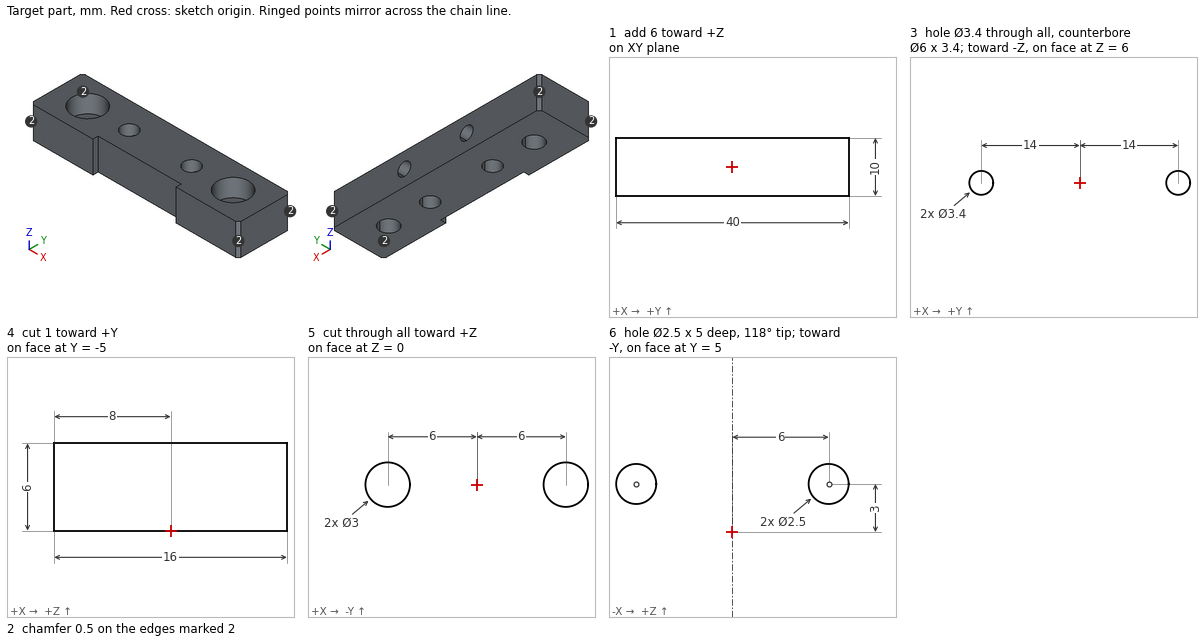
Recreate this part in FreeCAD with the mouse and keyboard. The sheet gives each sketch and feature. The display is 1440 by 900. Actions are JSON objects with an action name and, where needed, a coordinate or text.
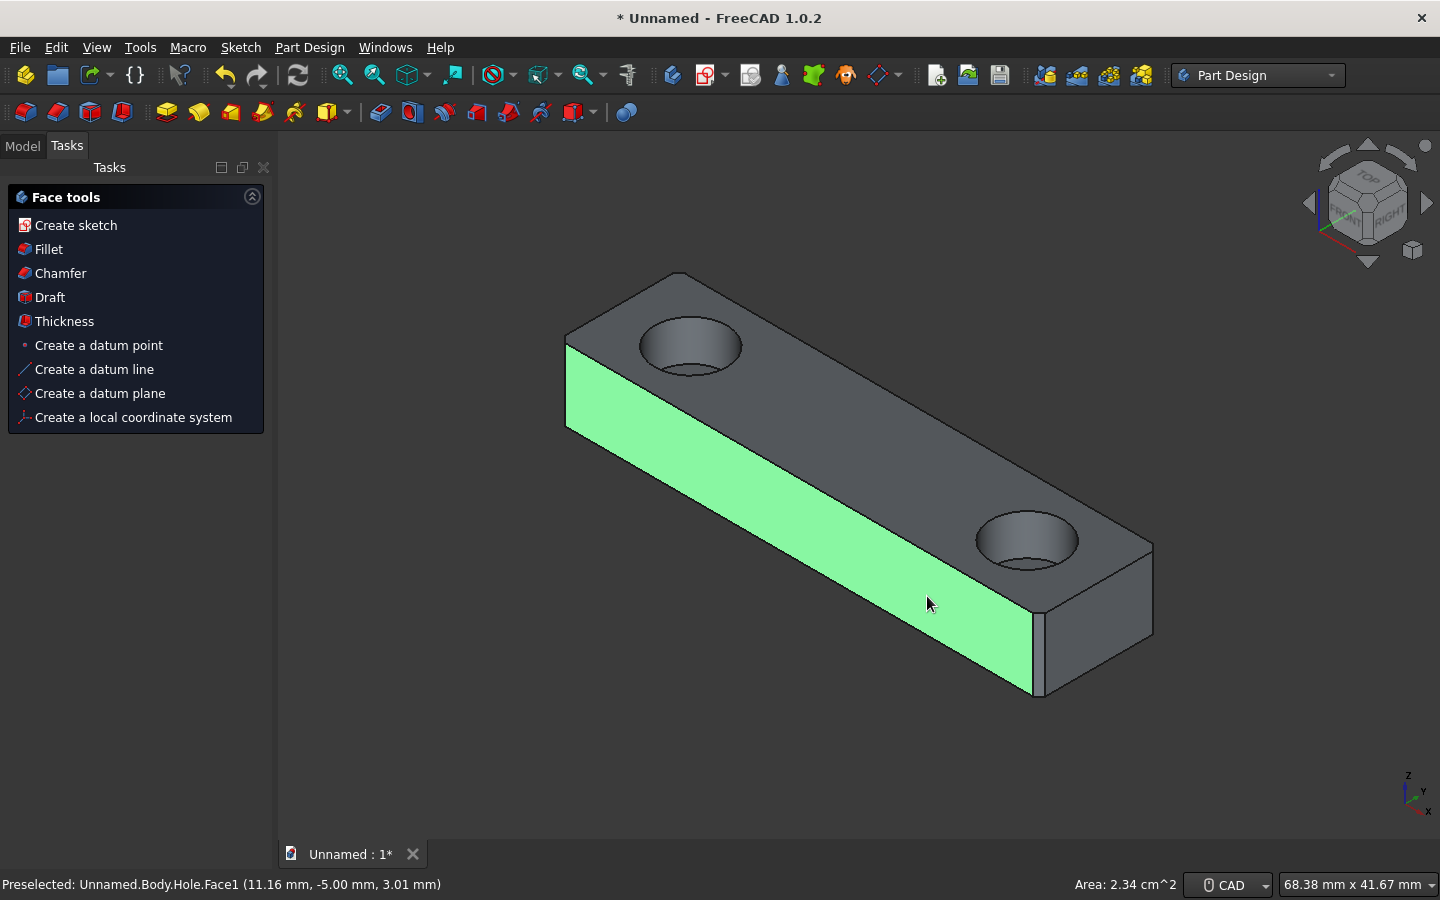
{"action": "left_click", "coordinate": [706, 76]}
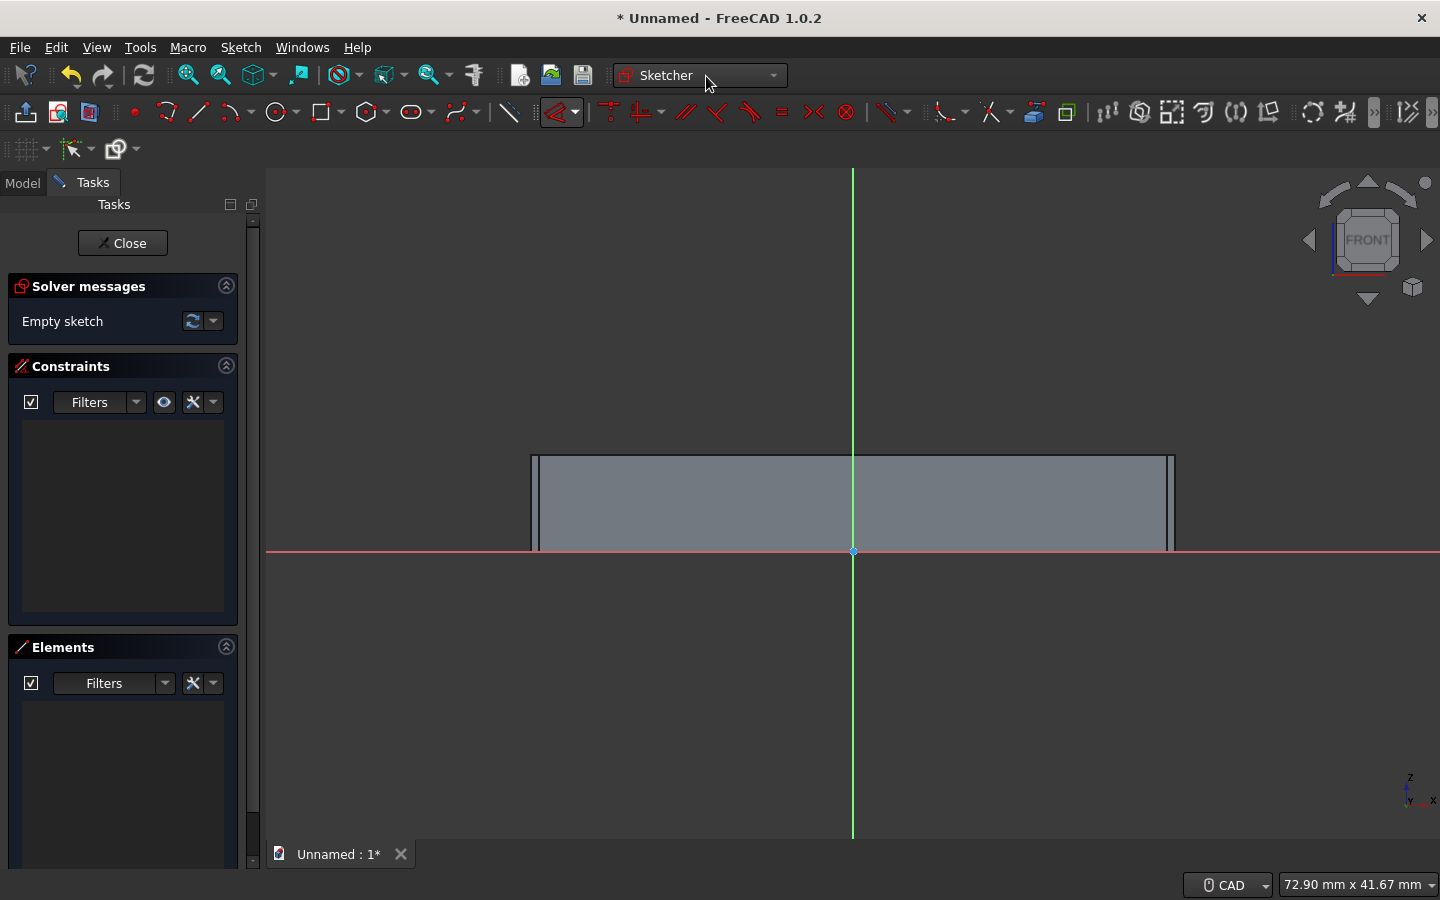
{"action": "scroll", "coordinate": [893, 503], "scroll_direction": "up", "scroll_amount": 5}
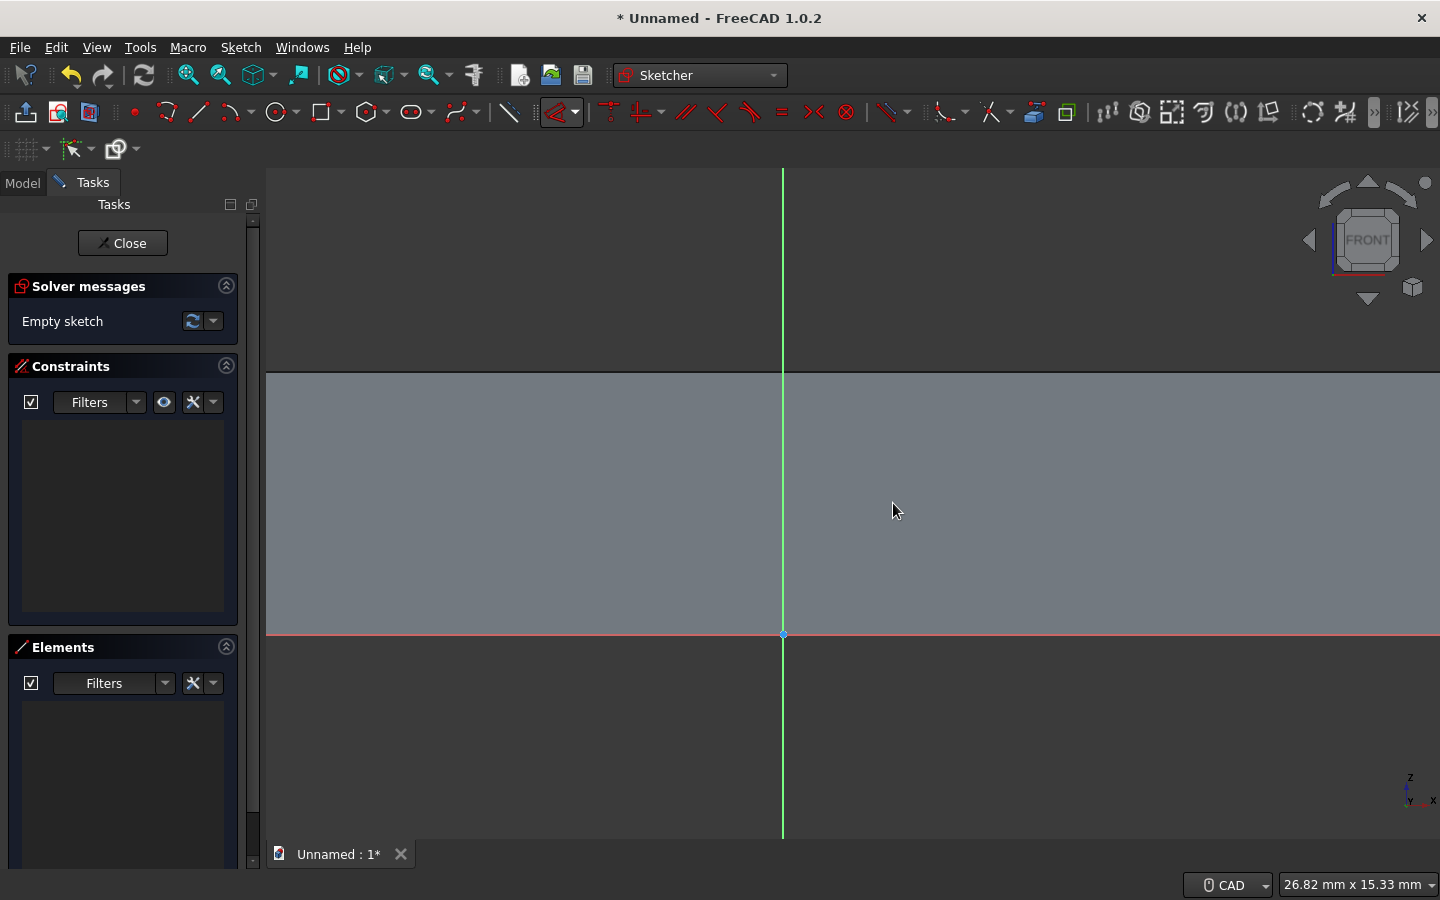
{"action": "left_click", "coordinate": [322, 112]}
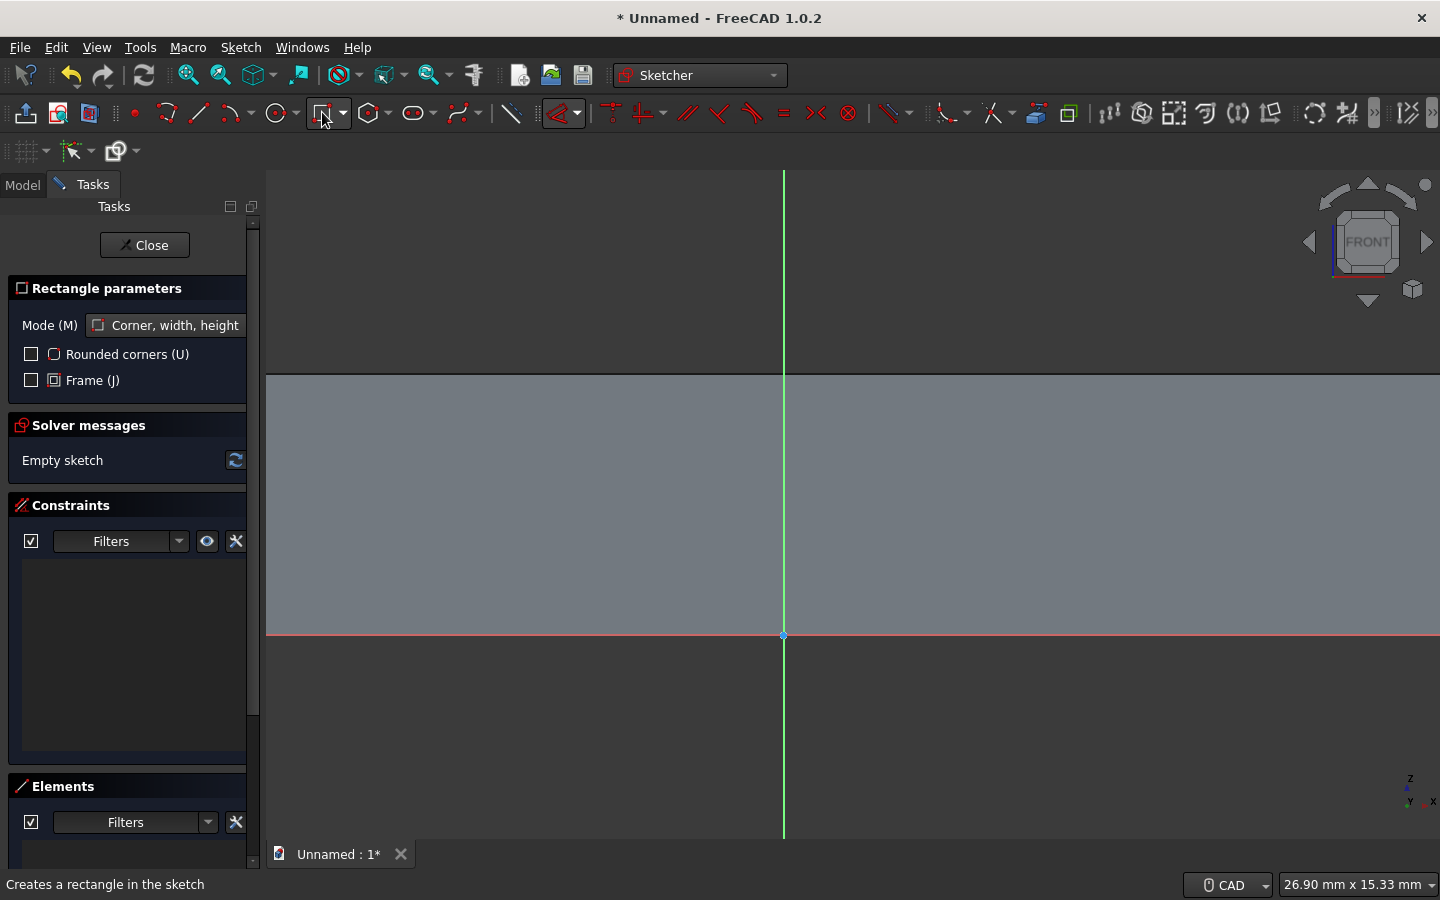
{"action": "left_click", "coordinate": [434, 374]}
{"action": "left_click", "coordinate": [1133, 635]}
{"action": "key", "text": "Escape"}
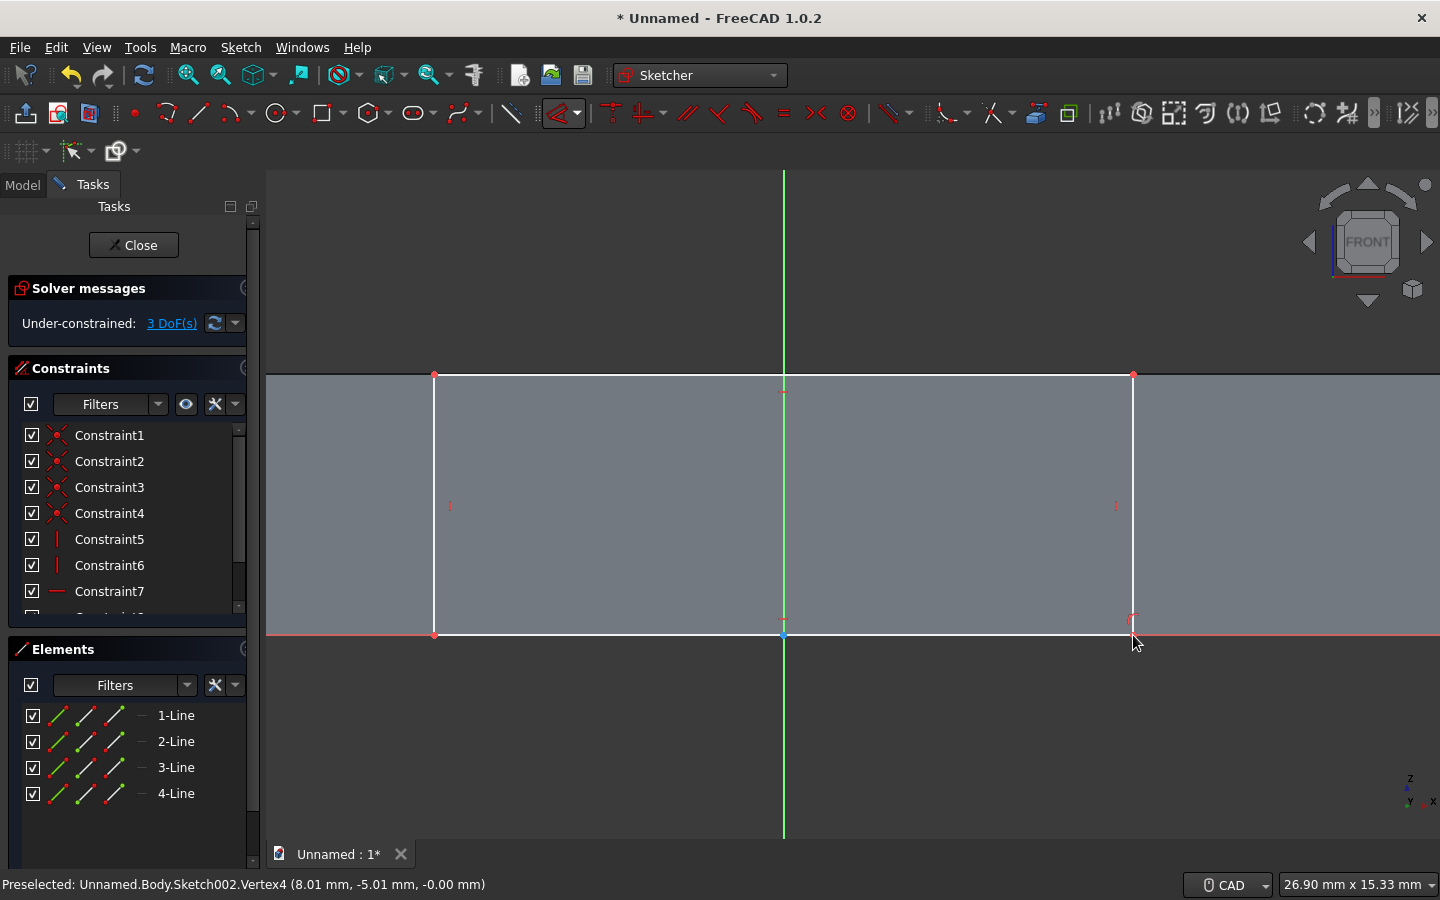
{"action": "left_click", "coordinate": [434, 453]}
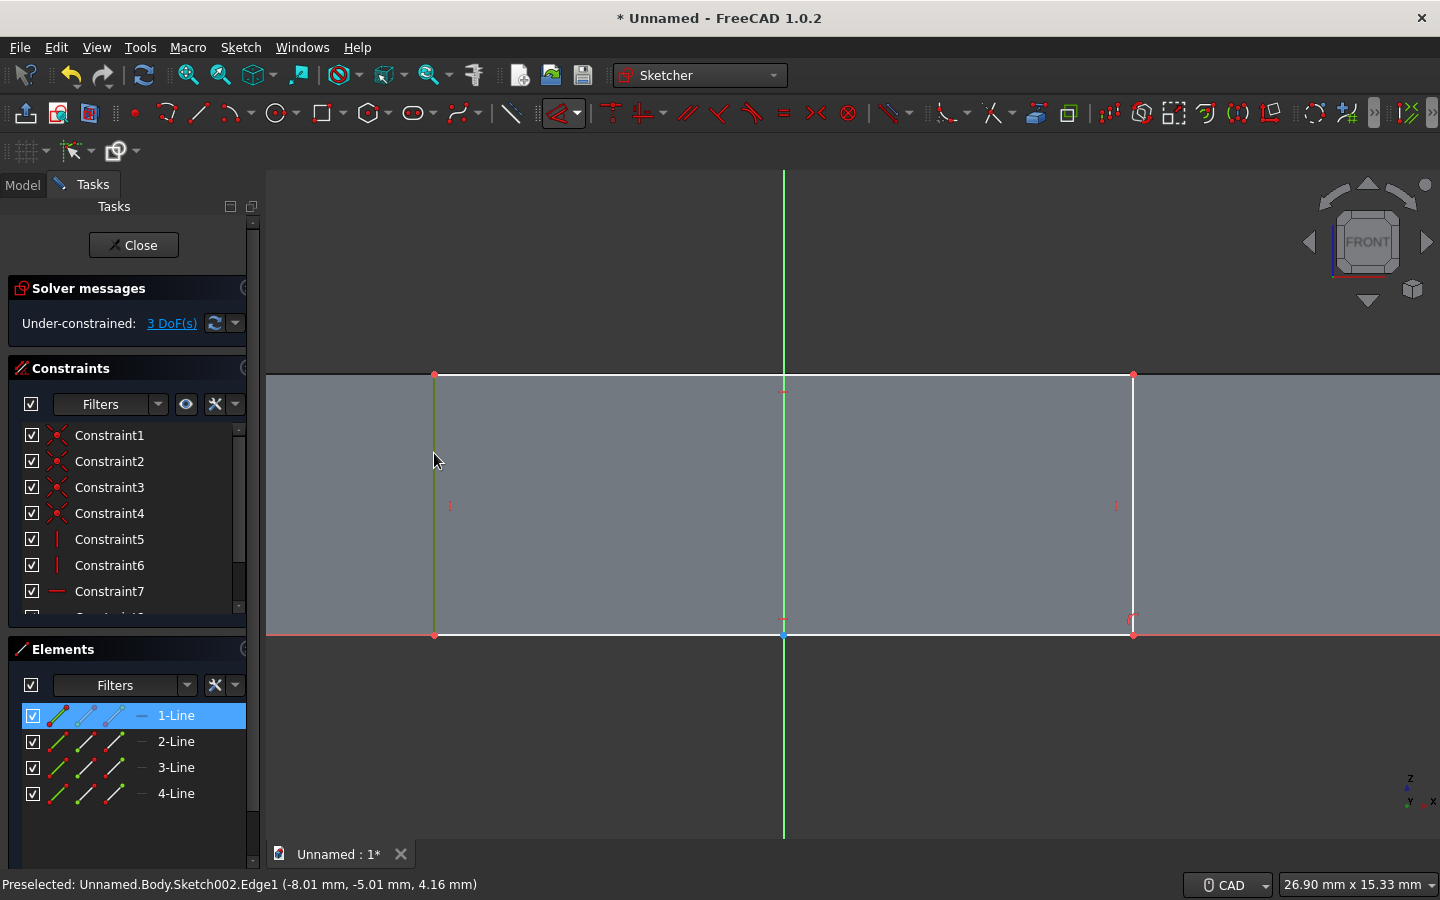
{"action": "key", "text": "i"}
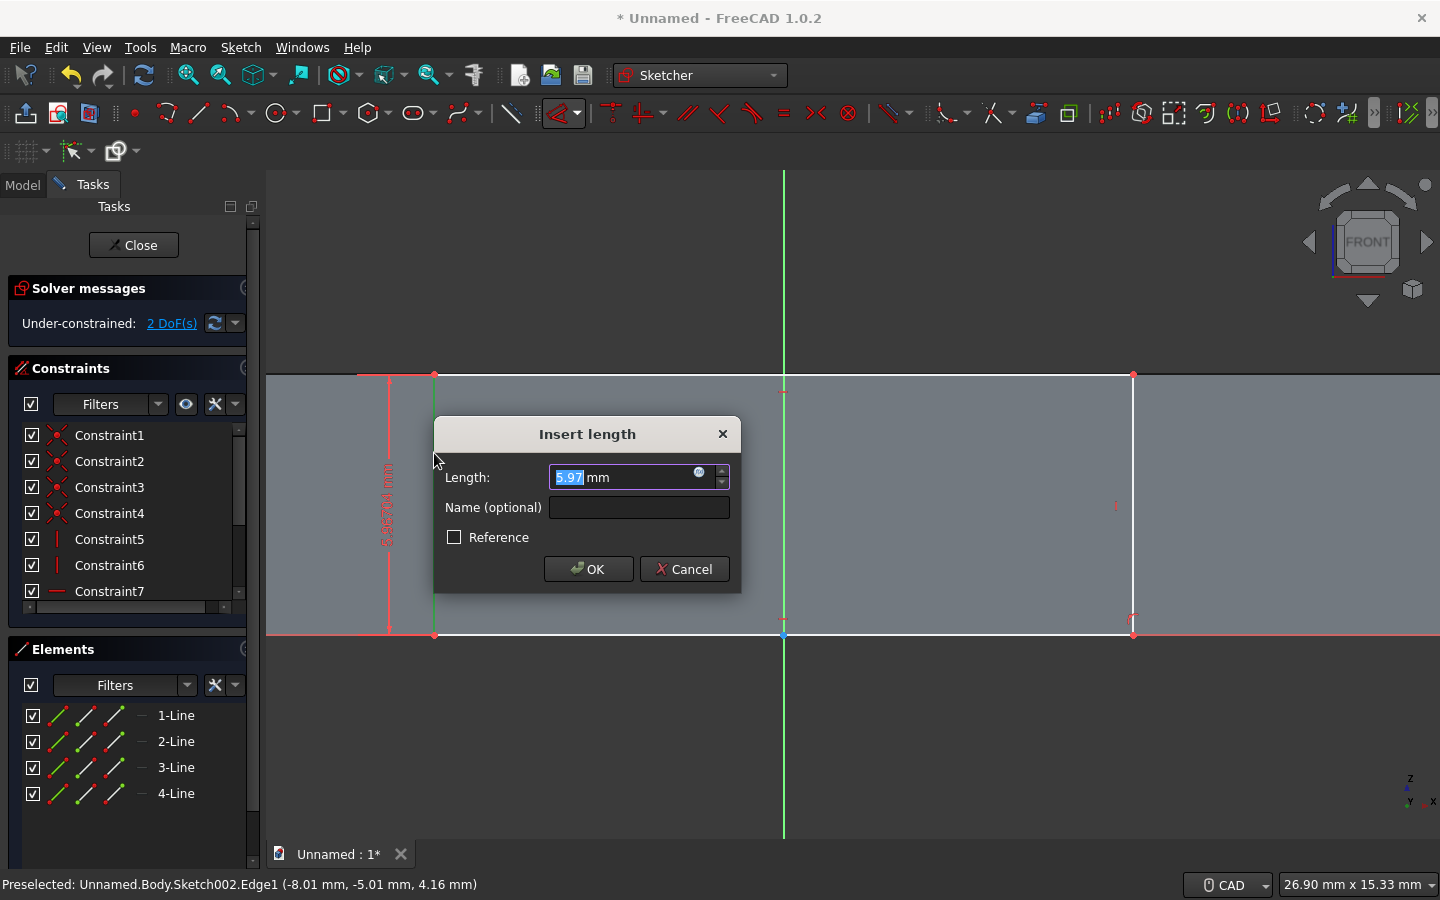
{"action": "type", "text": "6"}
{"action": "key", "text": "Return"}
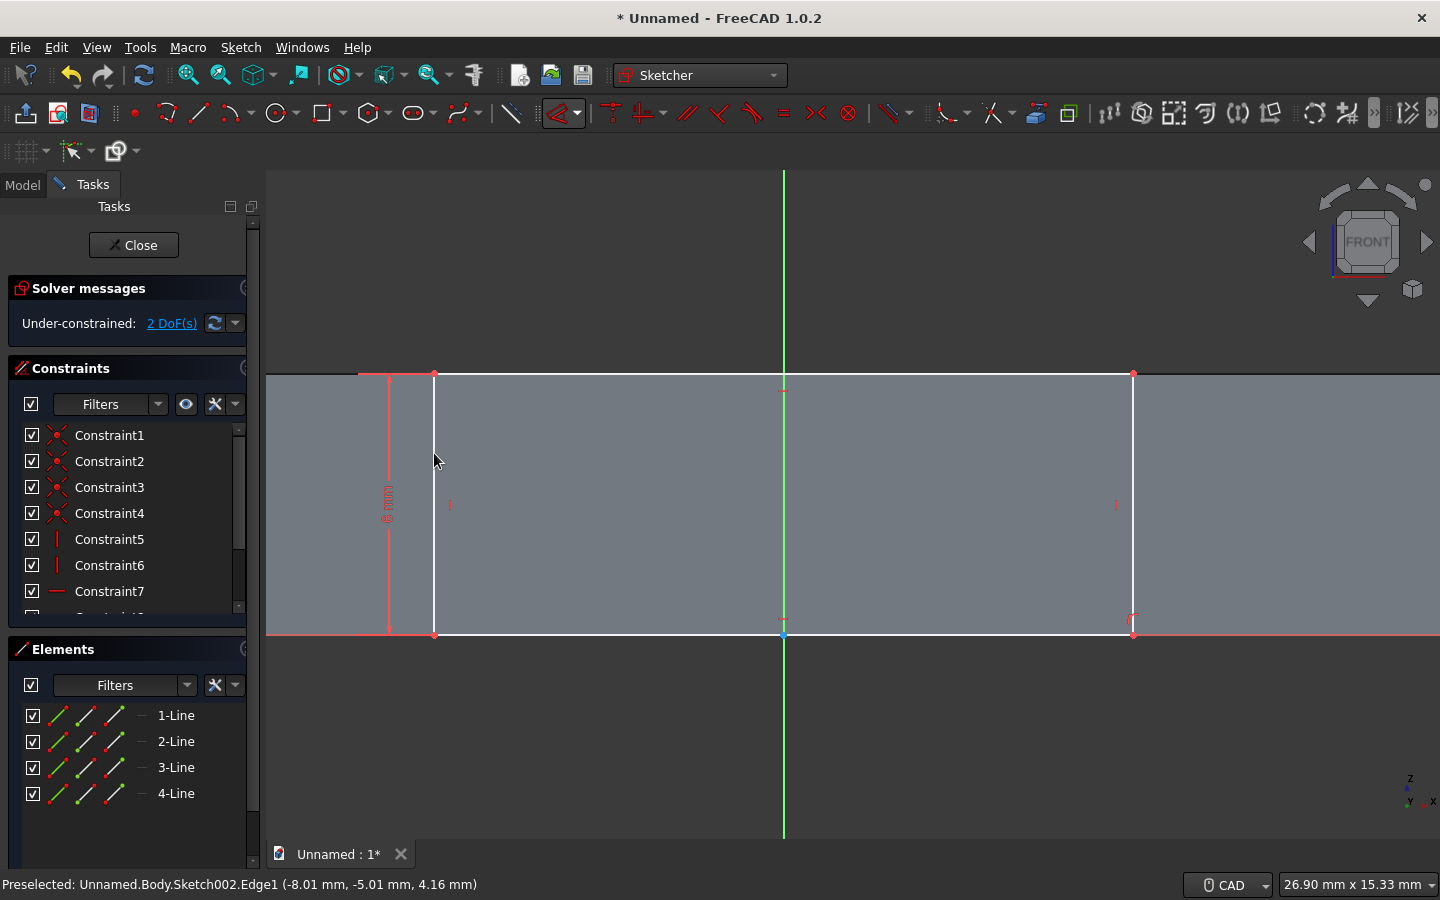
{"action": "left_click", "coordinate": [644, 635]}